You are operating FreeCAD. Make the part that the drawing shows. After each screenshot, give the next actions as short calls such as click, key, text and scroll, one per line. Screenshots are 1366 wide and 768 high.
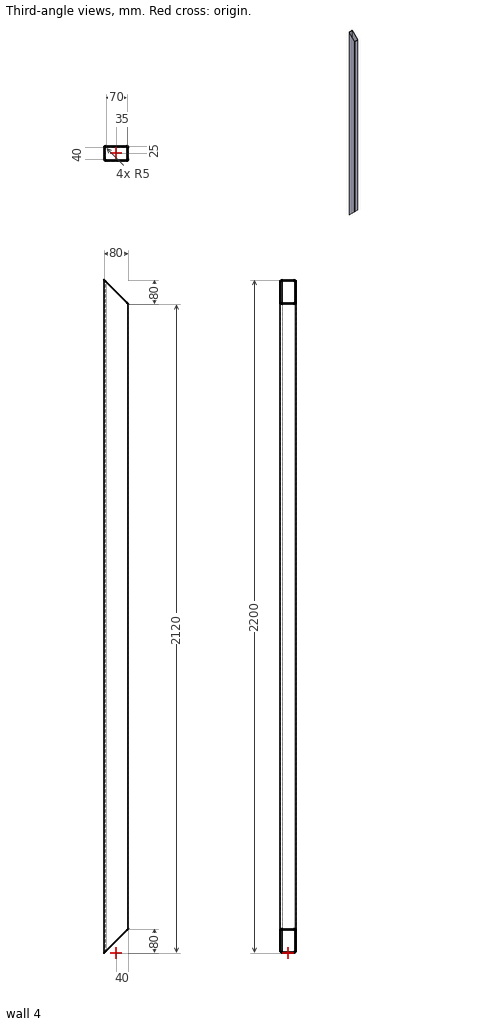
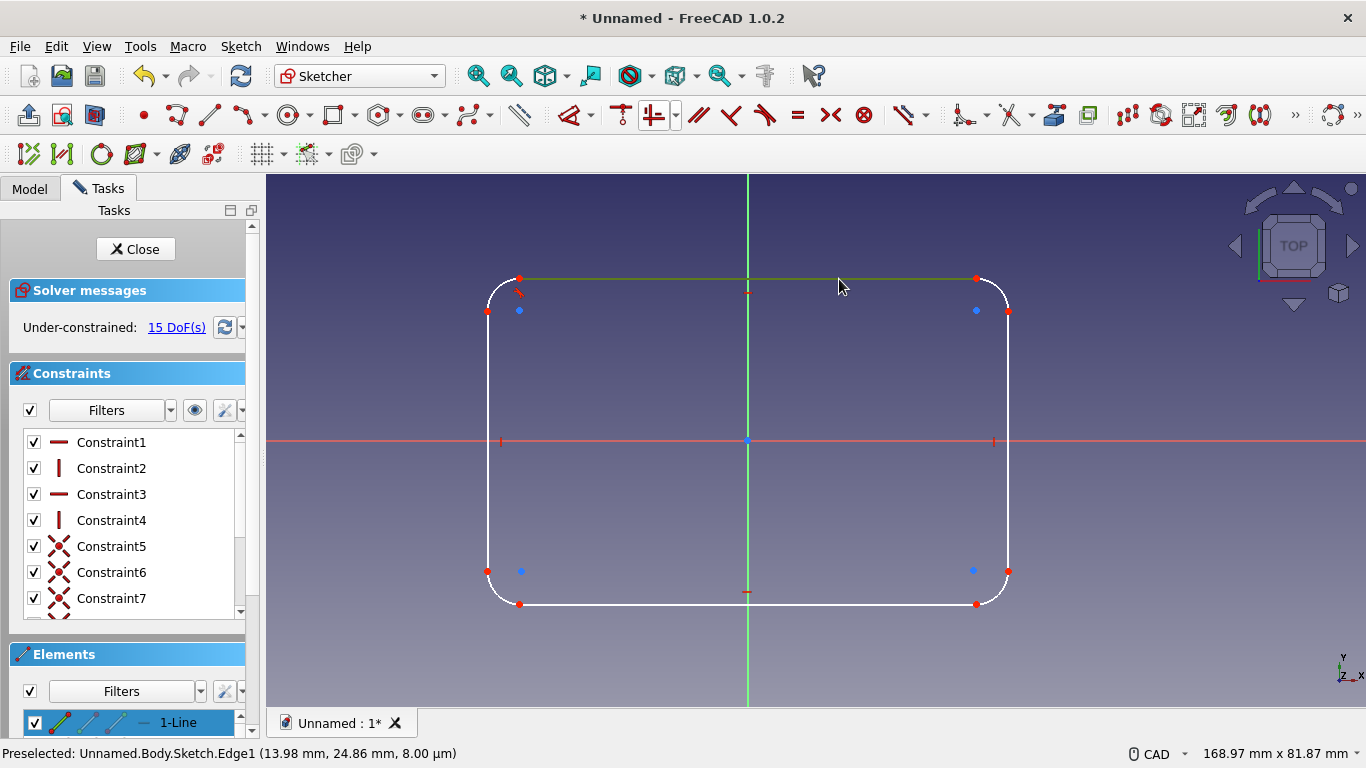
click(1005, 297)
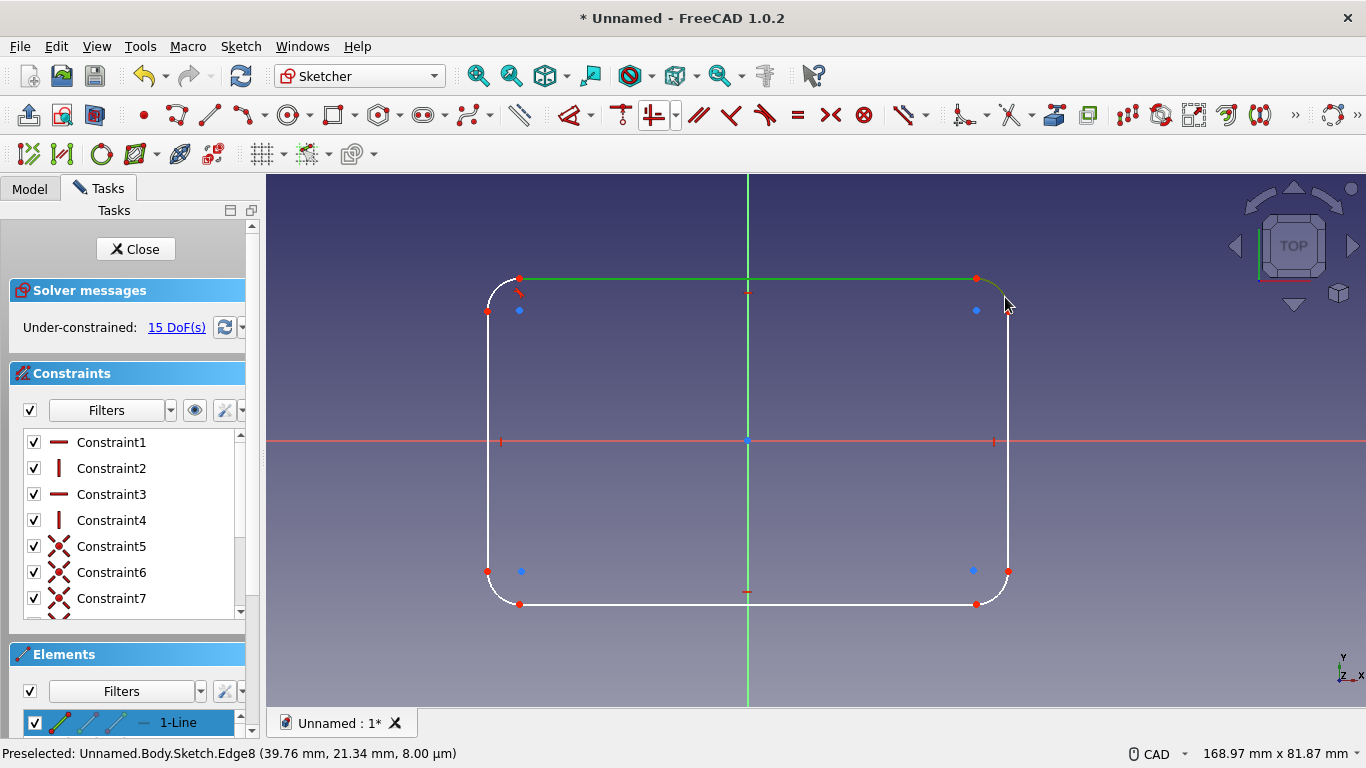
click(765, 116)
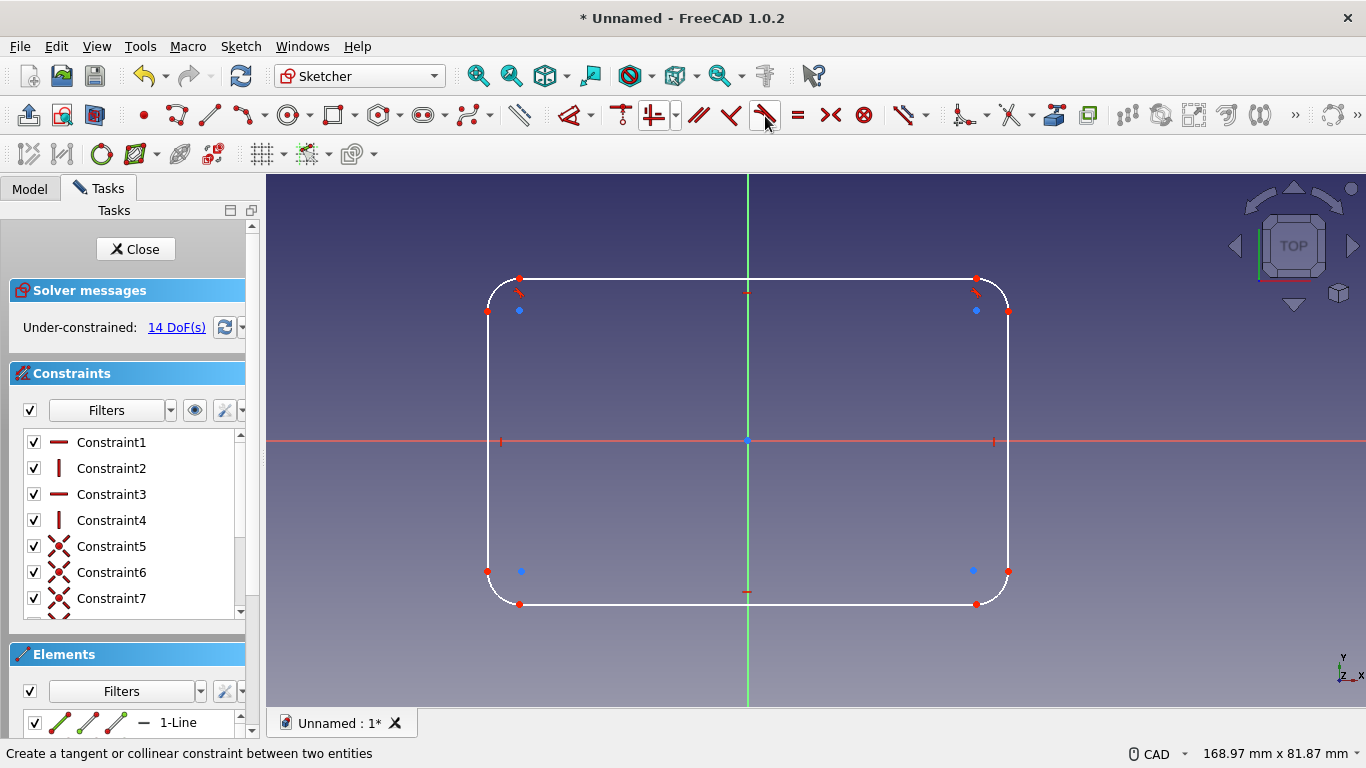
click(488, 390)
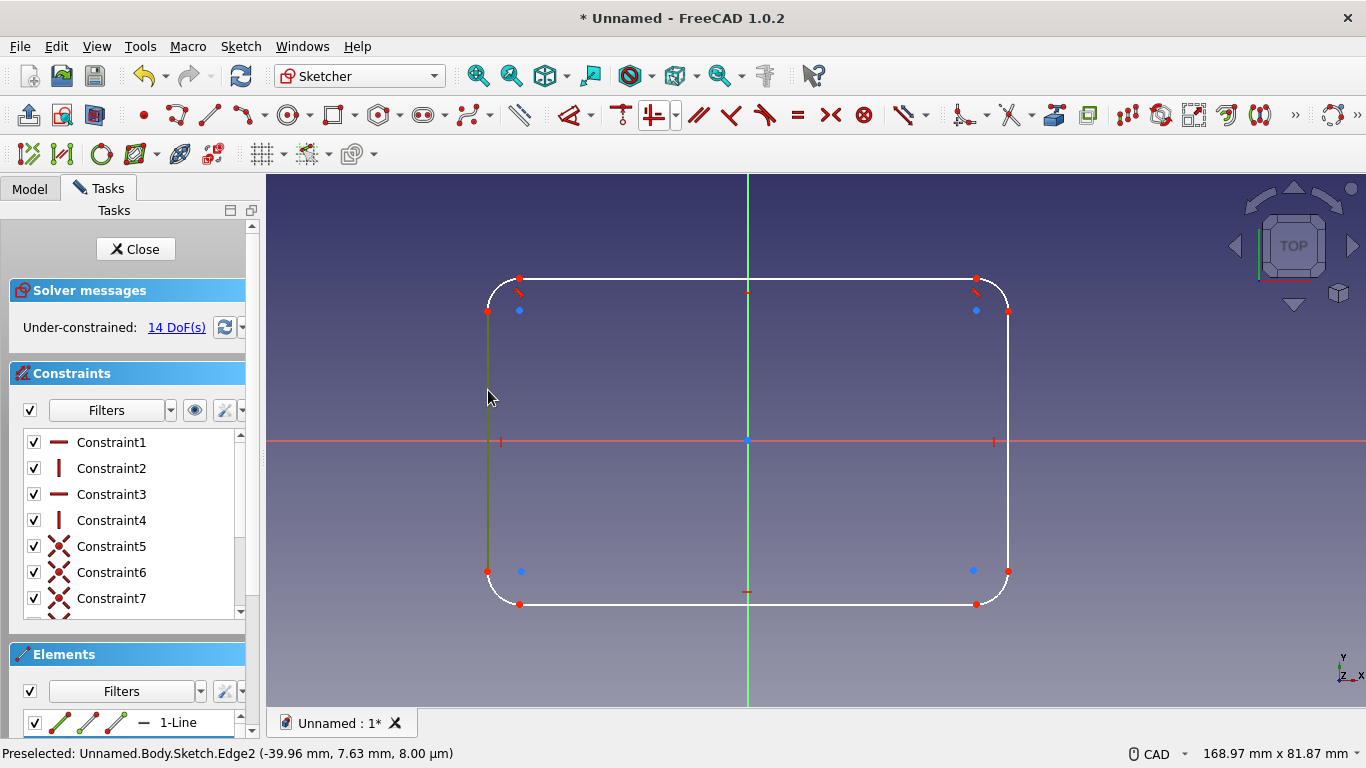
click(505, 282)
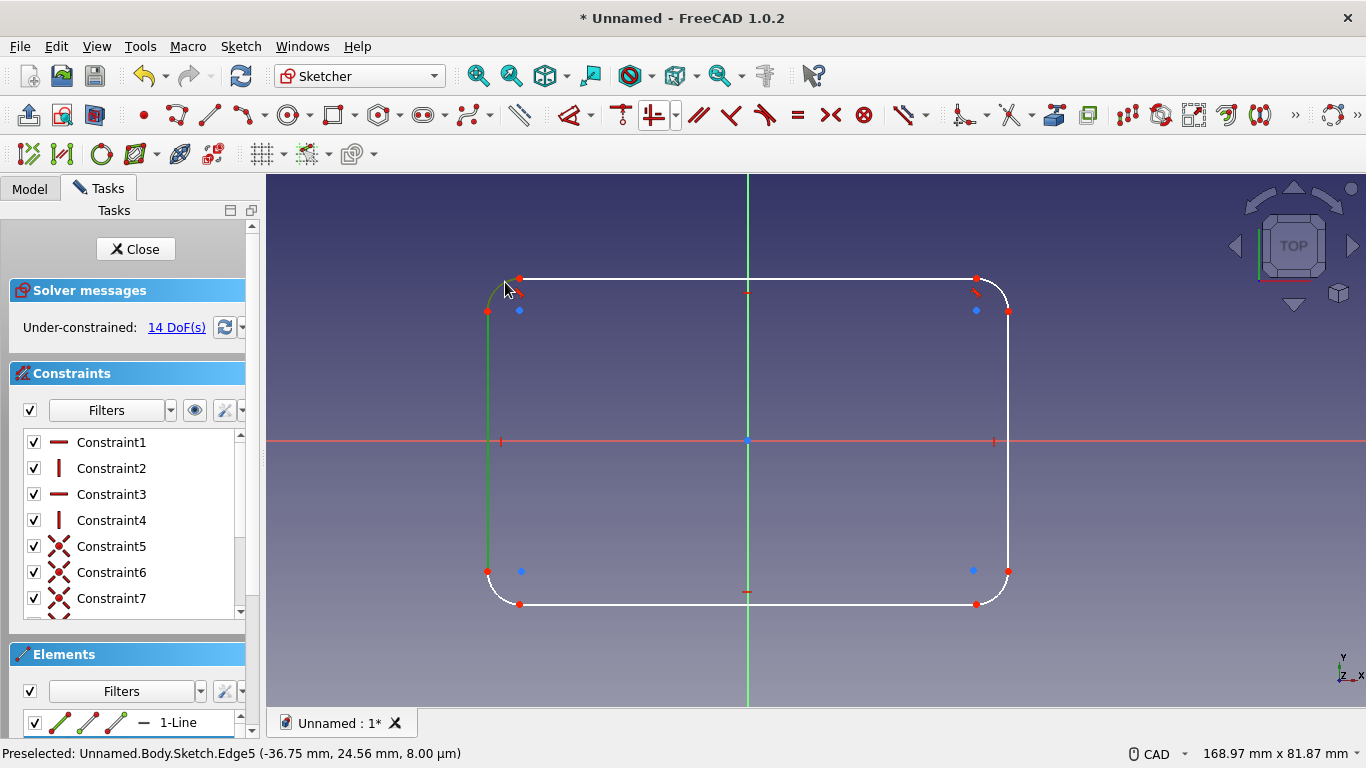
click(765, 116)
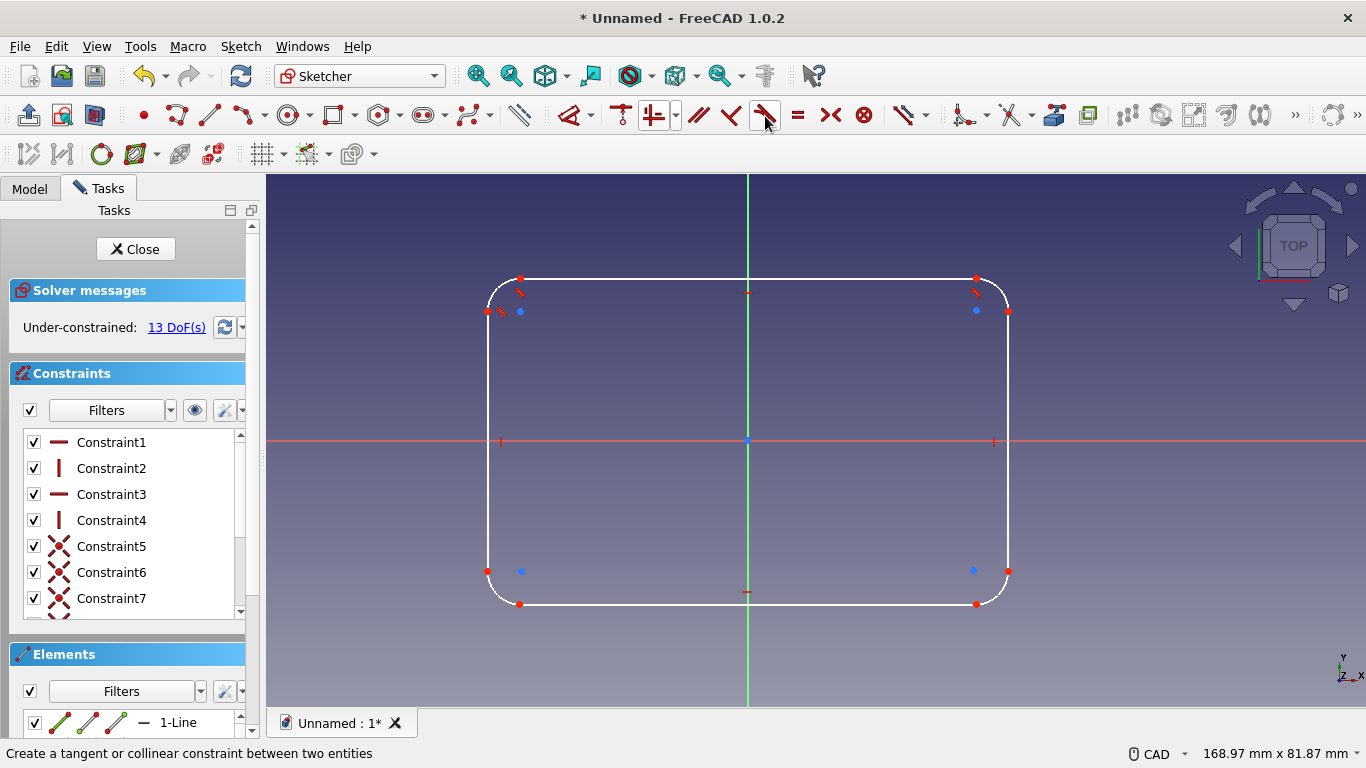
click(488, 390)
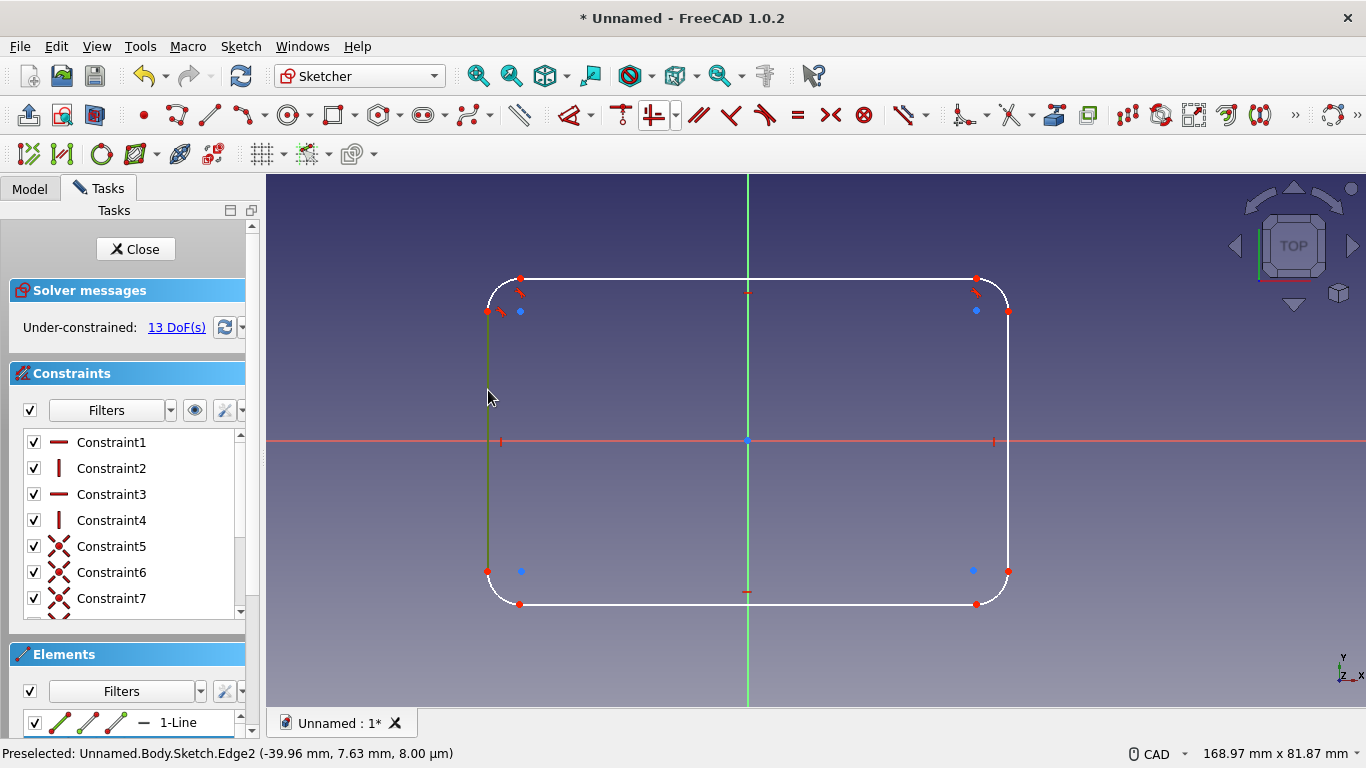
click(491, 586)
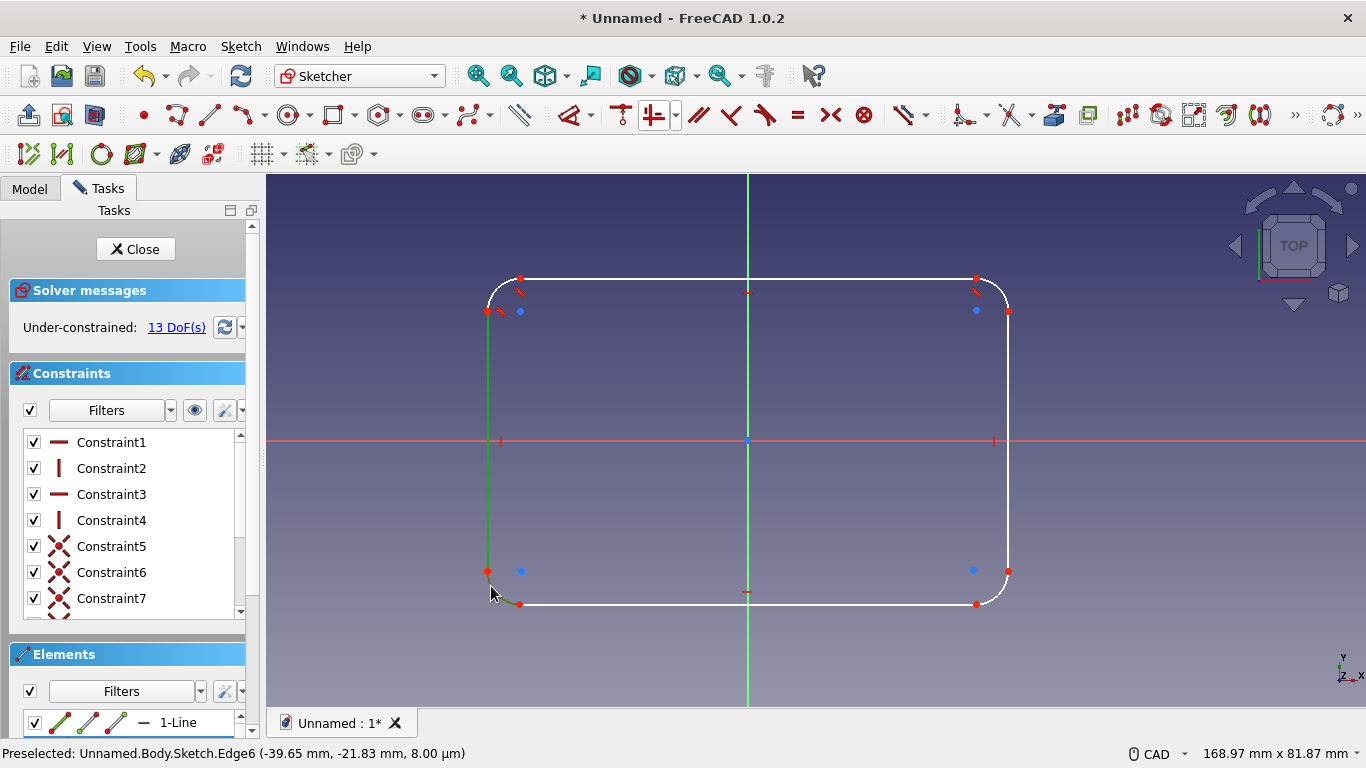
click(765, 116)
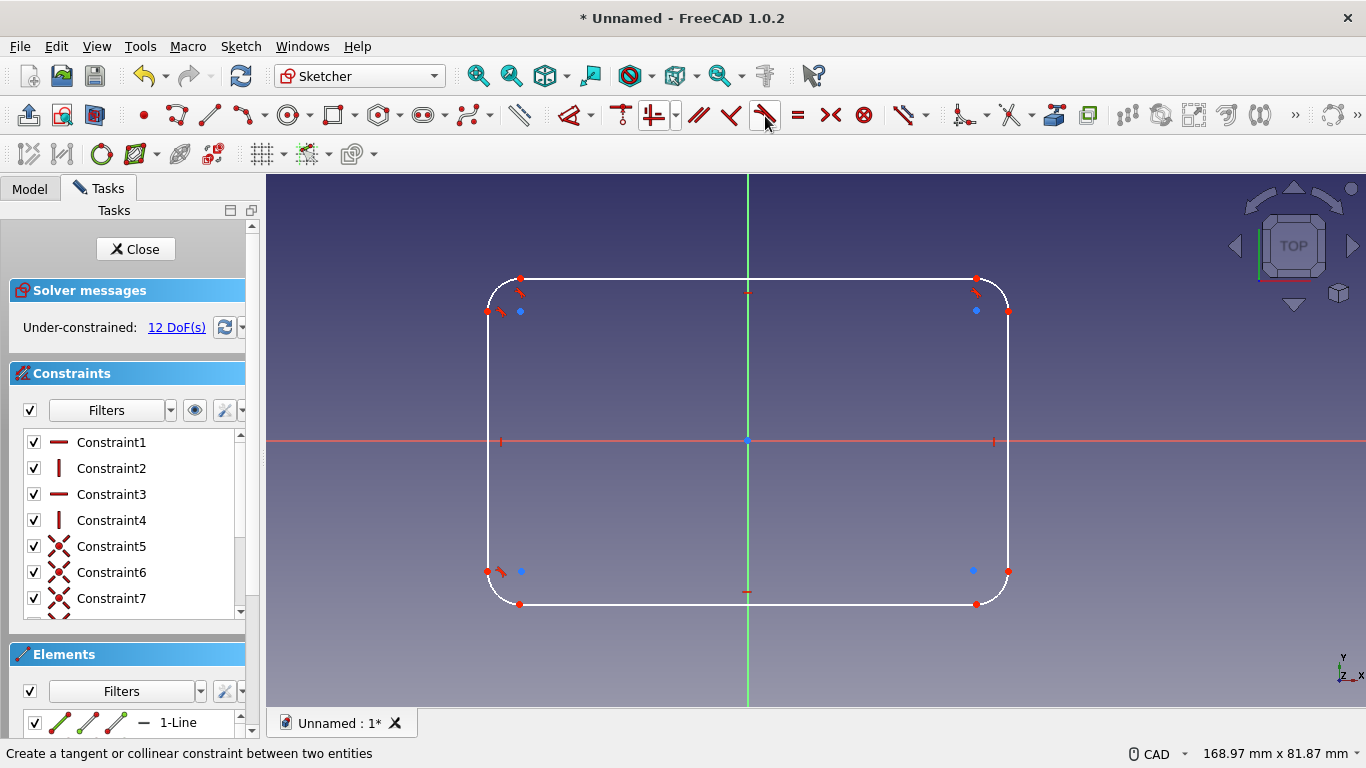
click(657, 605)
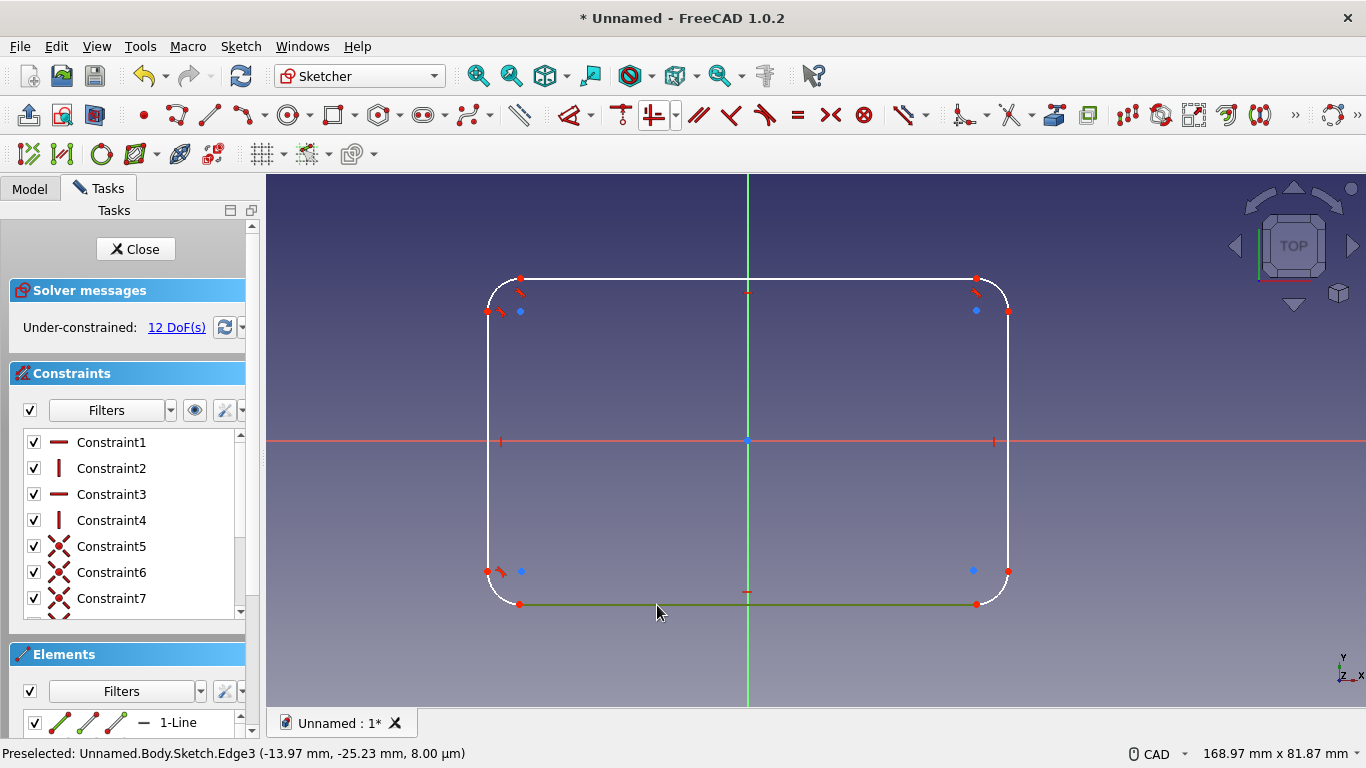
click(491, 586)